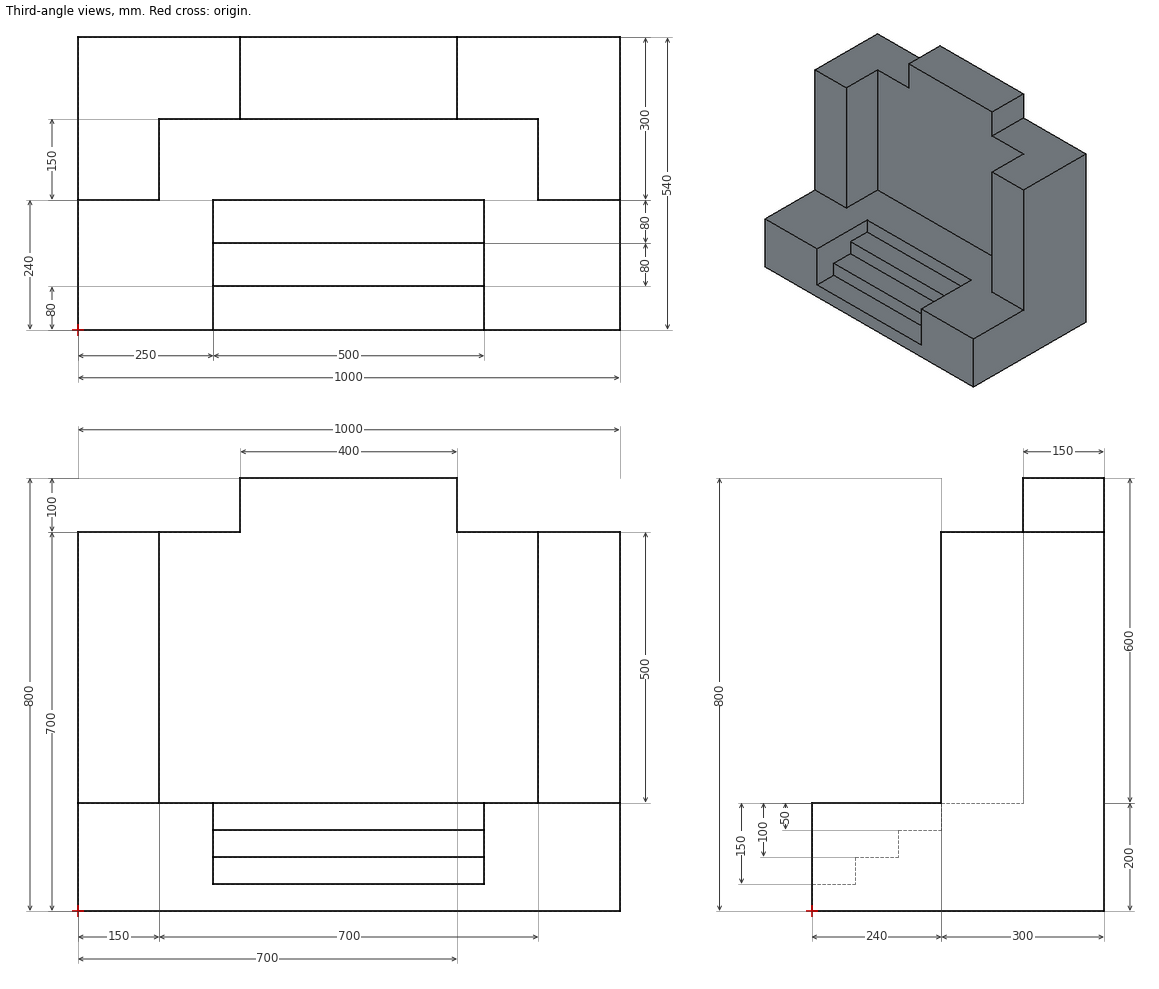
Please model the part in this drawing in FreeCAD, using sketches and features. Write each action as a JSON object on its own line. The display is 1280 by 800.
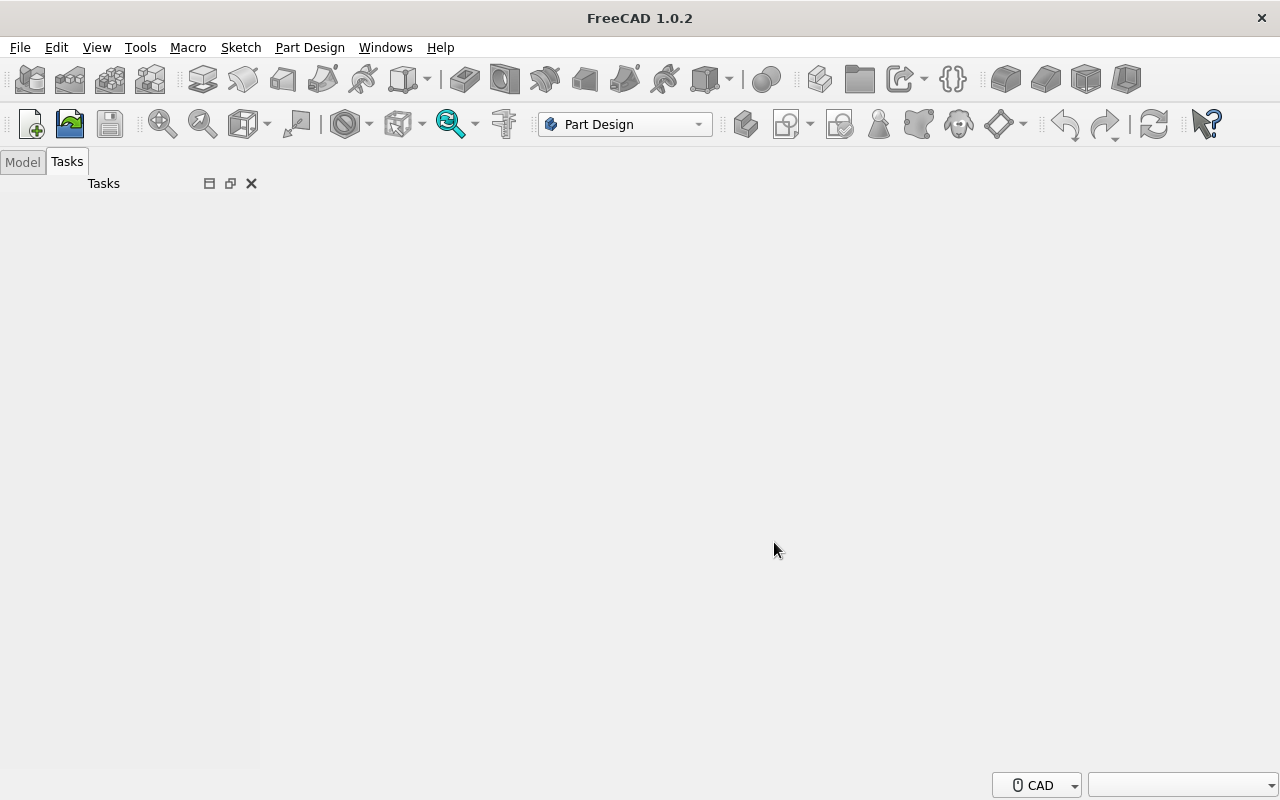
{"action": "left_click", "coordinate": [30, 124]}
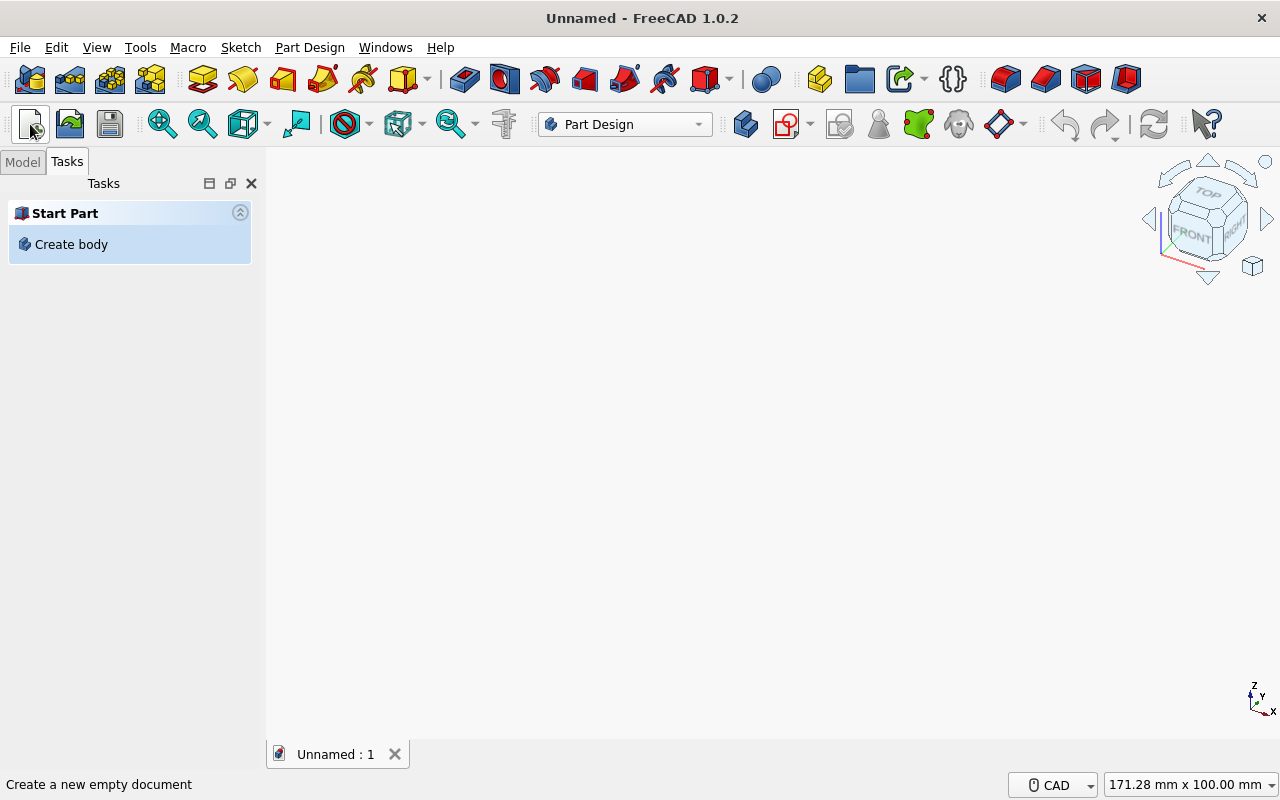
{"action": "left_click", "coordinate": [786, 124]}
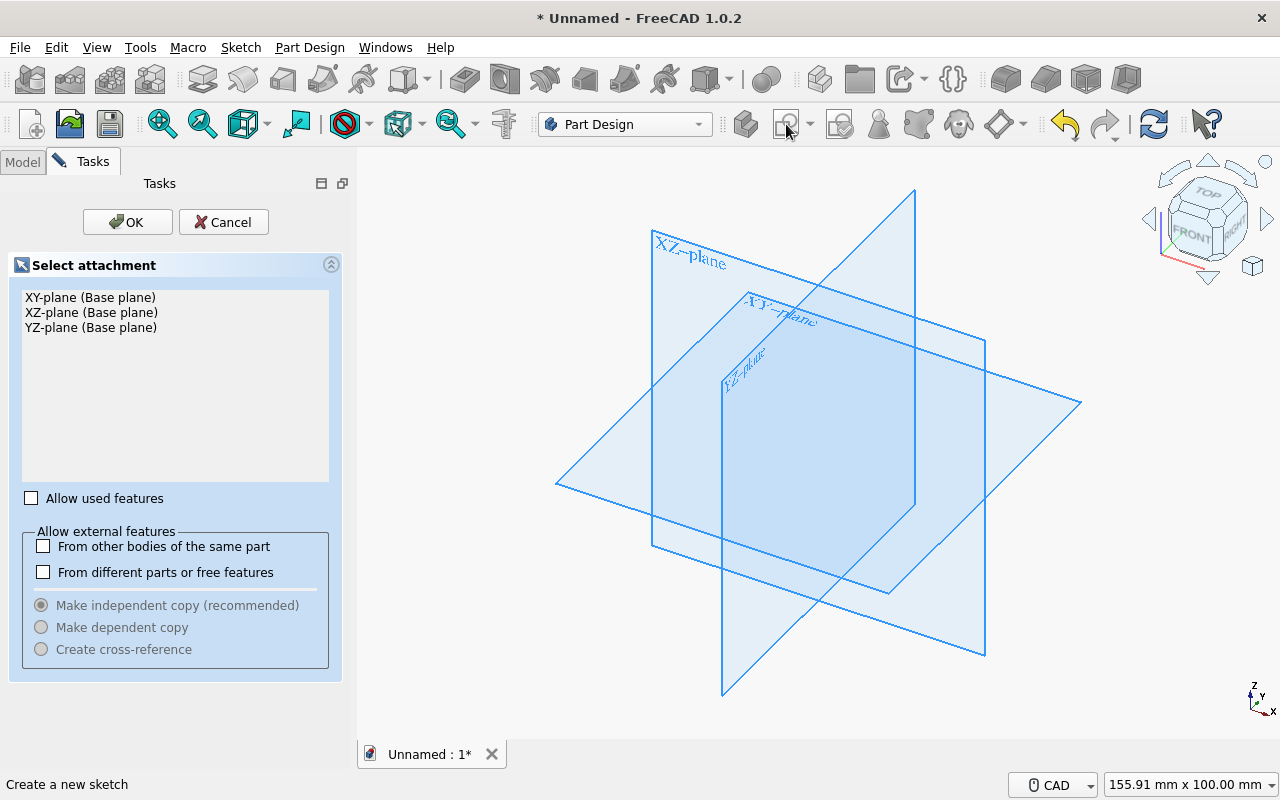
{"action": "left_click", "coordinate": [82, 298]}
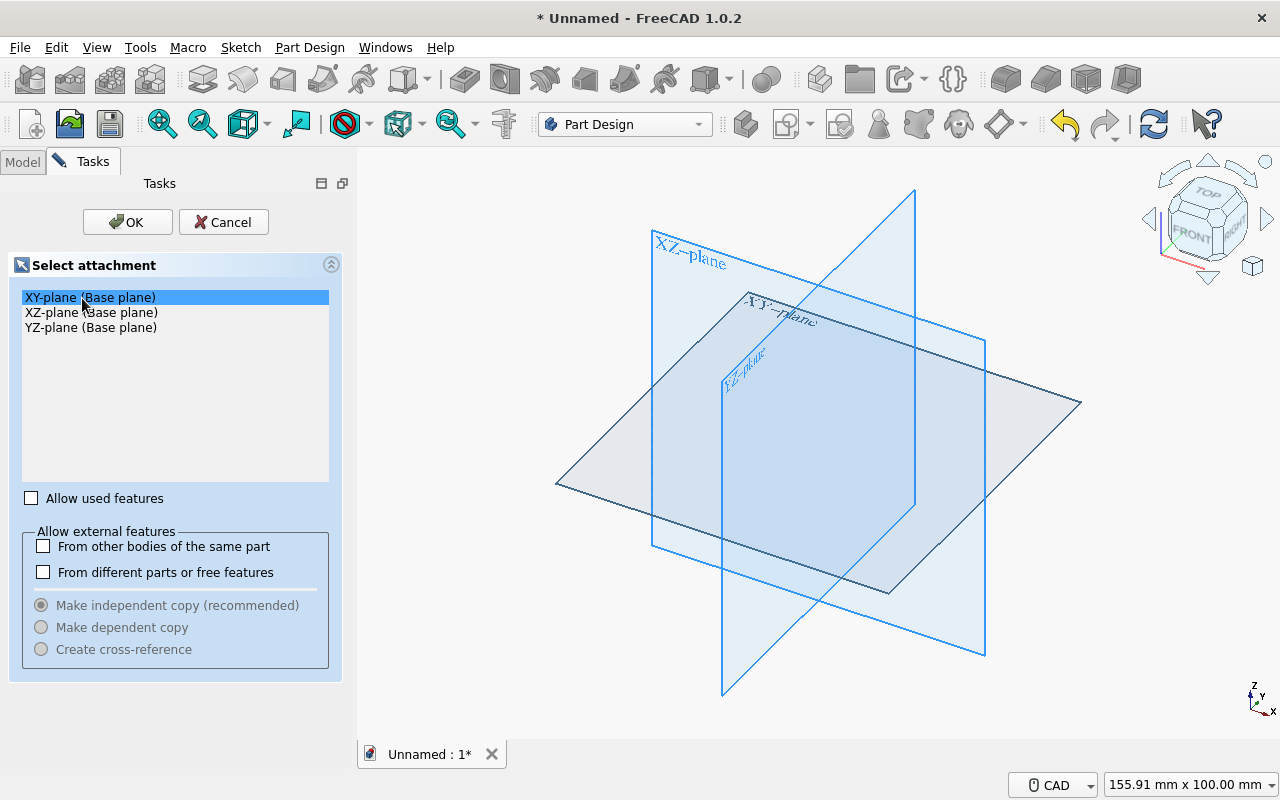
{"action": "left_click", "coordinate": [128, 222]}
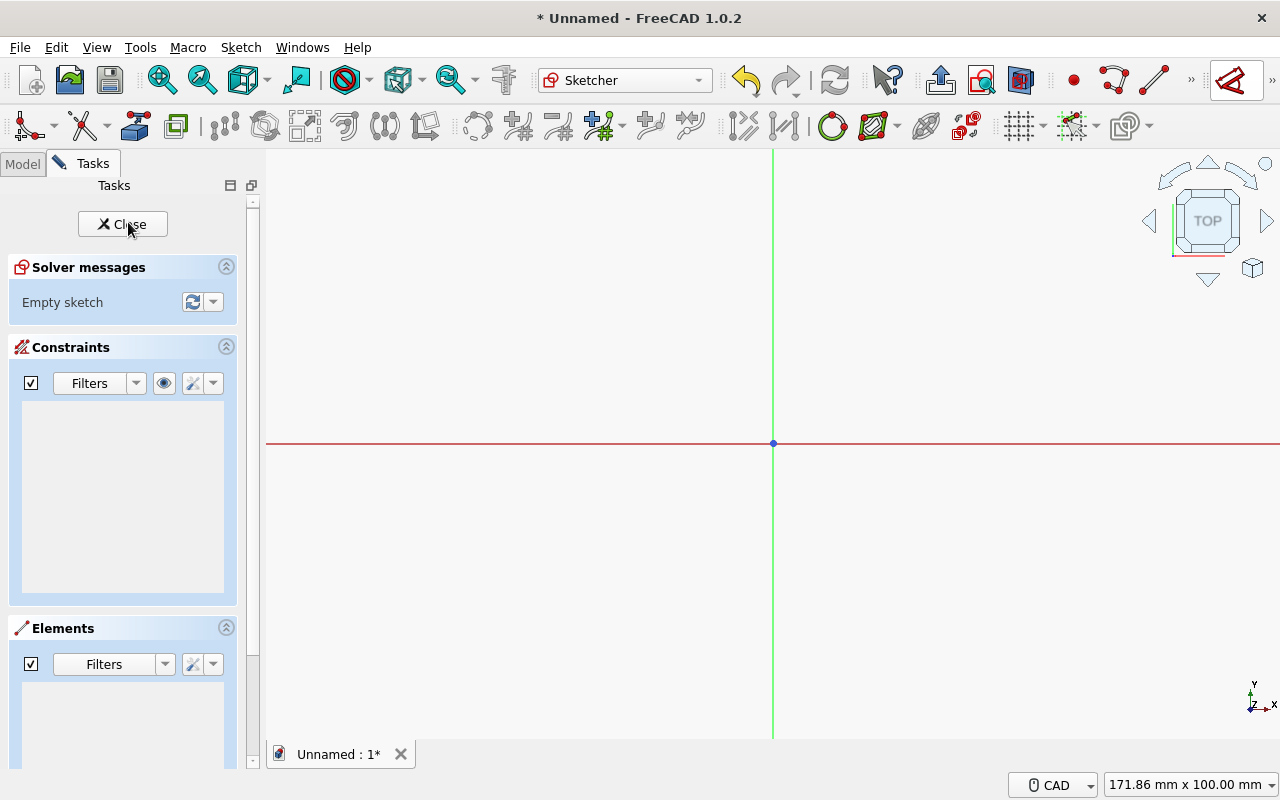
{"action": "scroll", "coordinate": [403, 603], "scroll_direction": "down", "scroll_amount": 12}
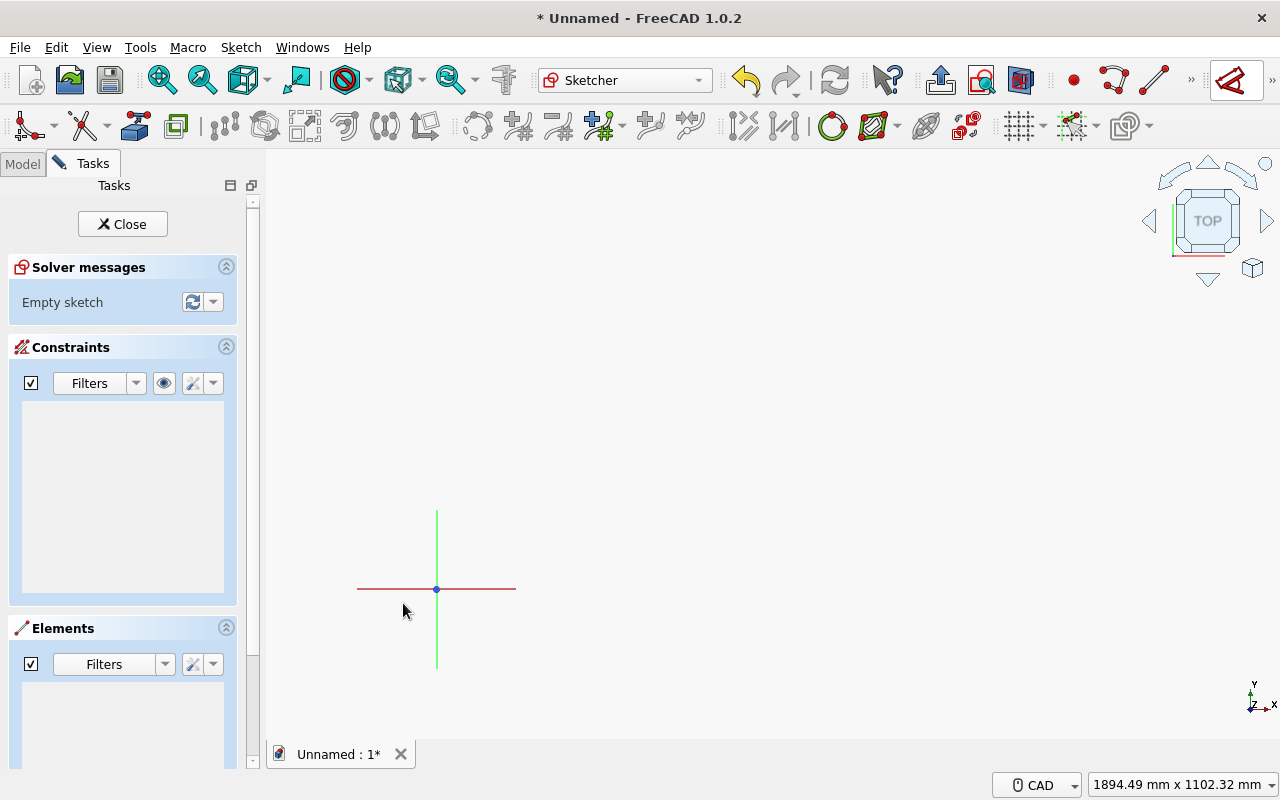
{"action": "key", "text": "g r"}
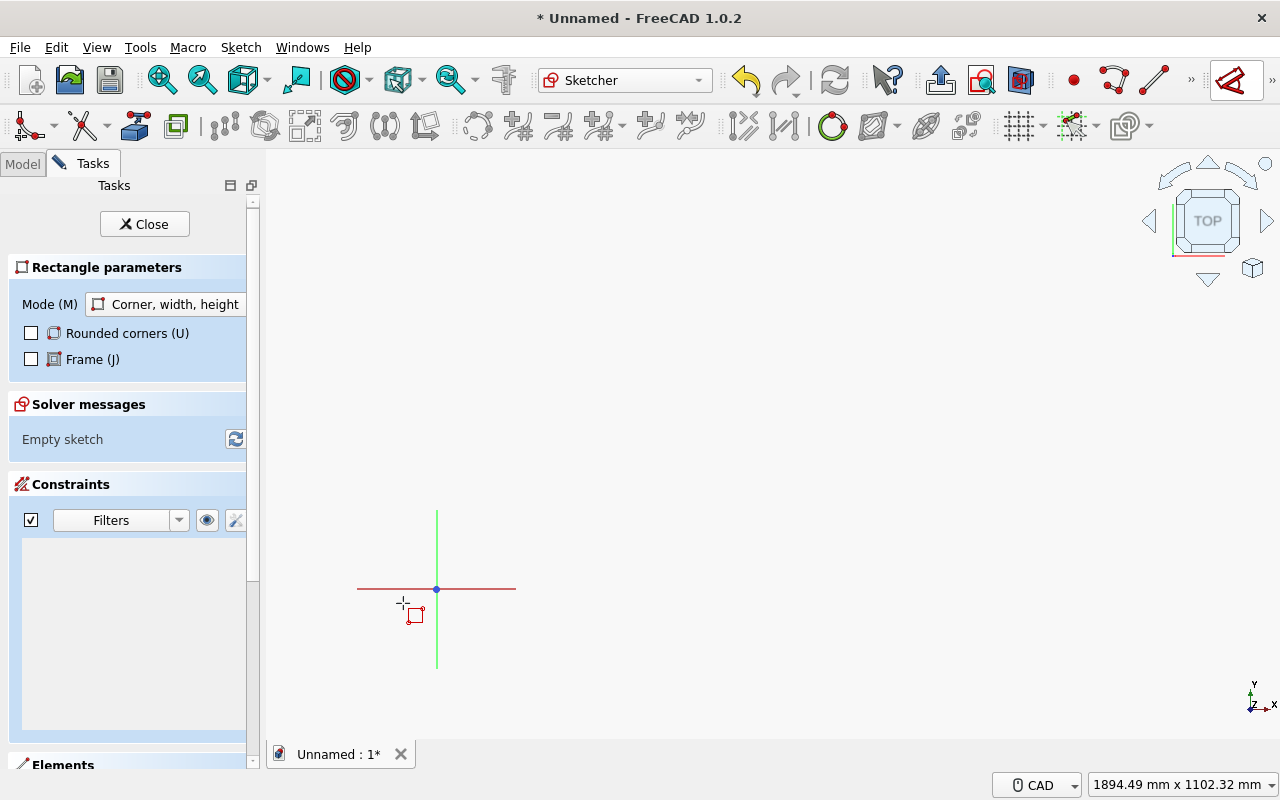
{"action": "left_click", "coordinate": [437, 589]}
{"action": "mouse_move", "coordinate": [972, 300]}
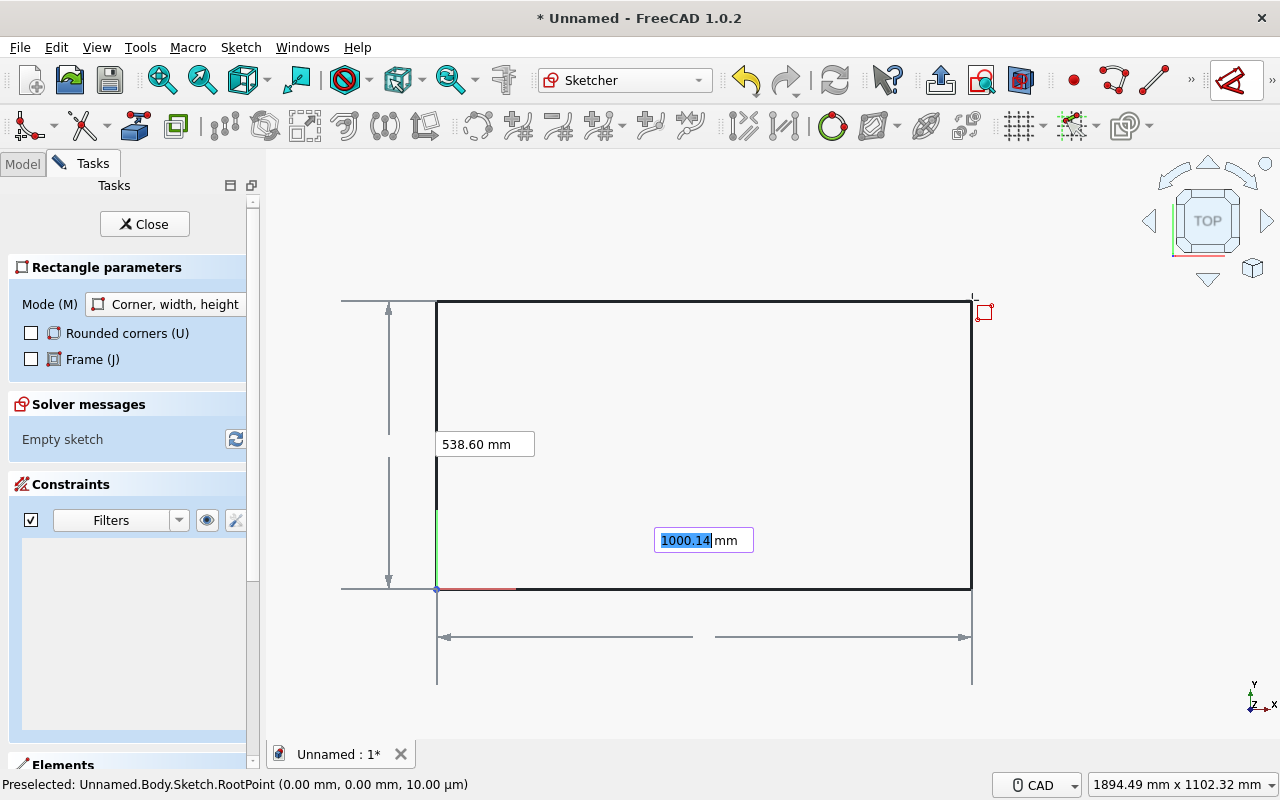
{"action": "type", "text": "1000"}
{"action": "key", "text": "Tab"}
{"action": "type", "text": "540"}
{"action": "key", "text": "Return"}
{"action": "key", "text": "Escape"}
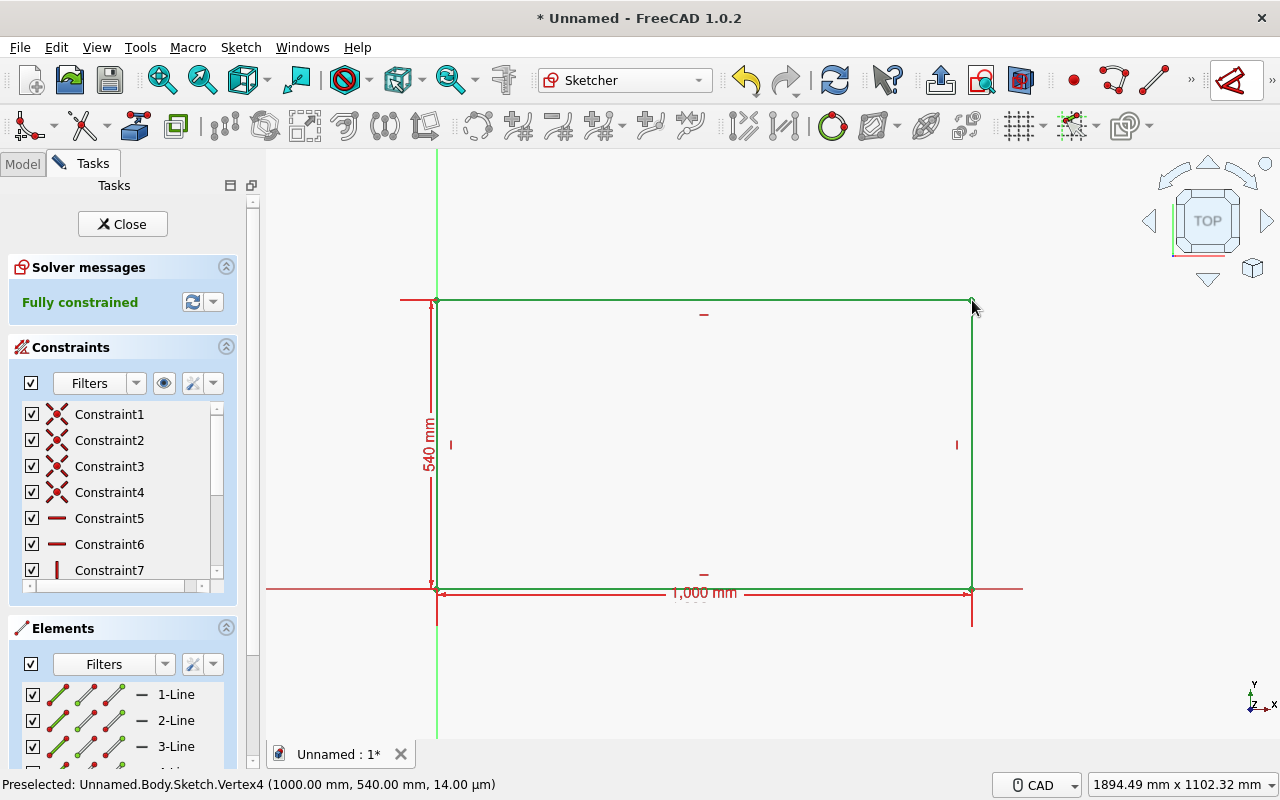
{"action": "left_click", "coordinate": [123, 224]}